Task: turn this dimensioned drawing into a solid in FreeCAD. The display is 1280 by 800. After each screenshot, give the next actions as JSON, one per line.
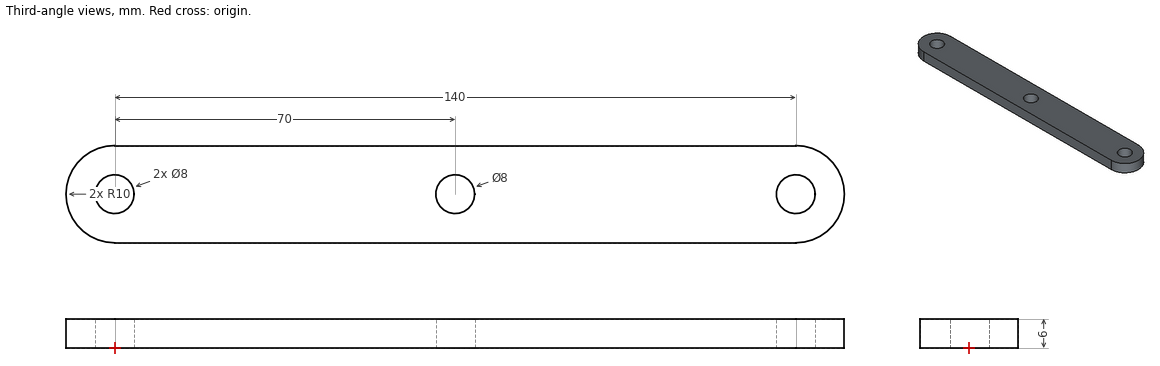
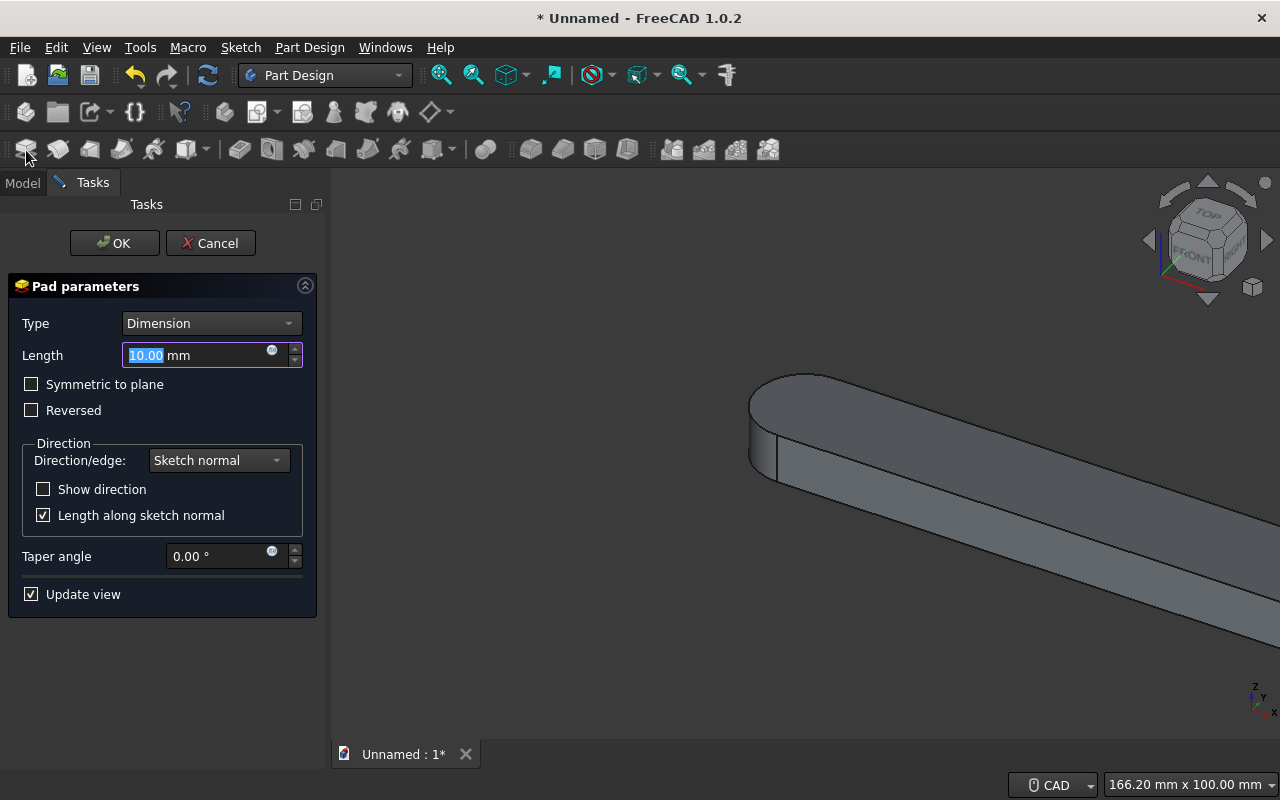
{"action": "type", "text": "6"}
{"action": "key", "text": "Tab"}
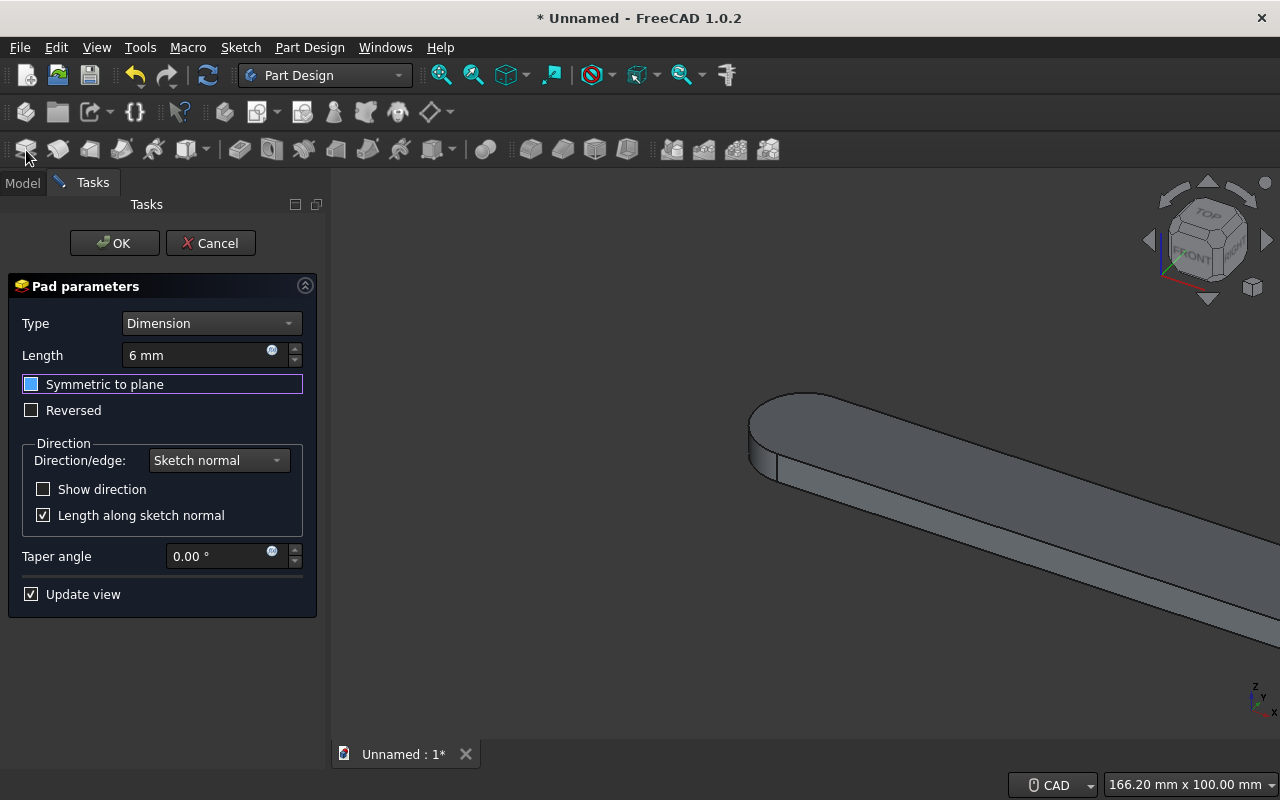
{"action": "left_click", "coordinate": [115, 243]}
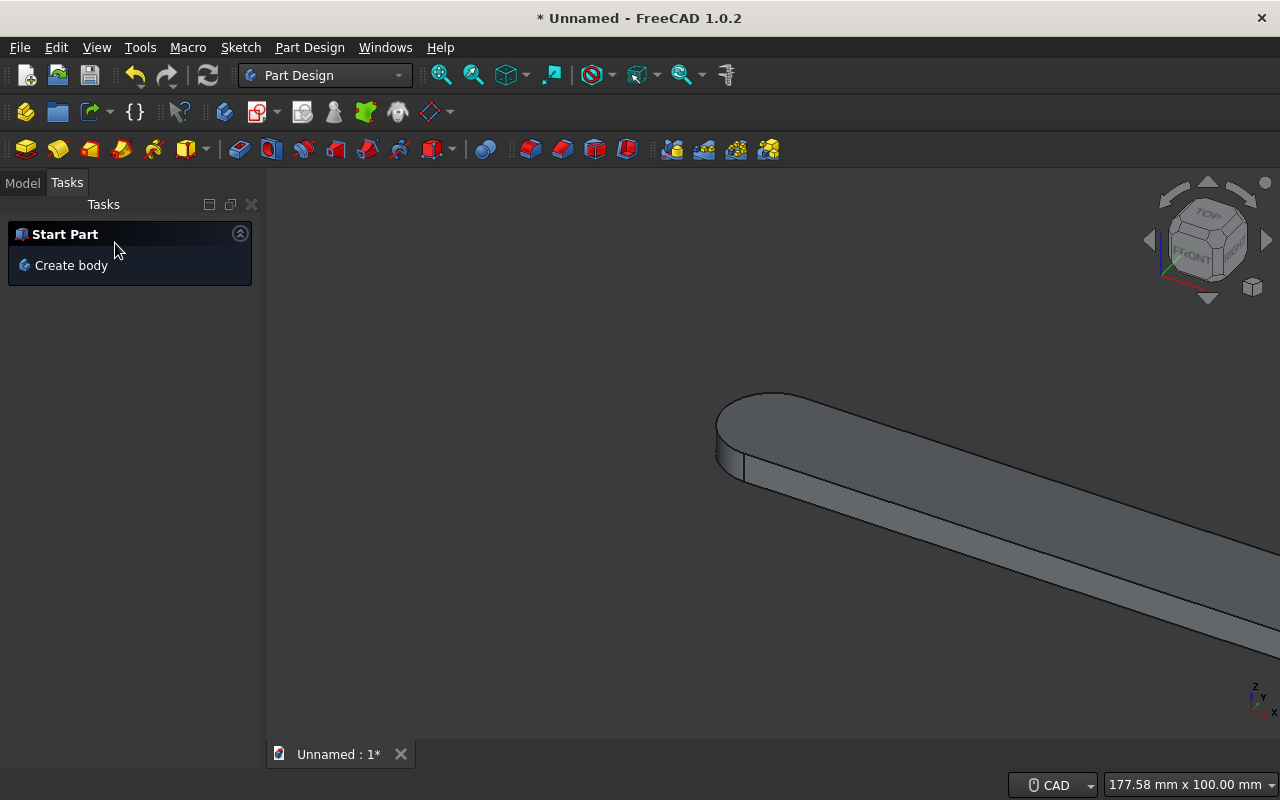
{"action": "left_click", "coordinate": [442, 76]}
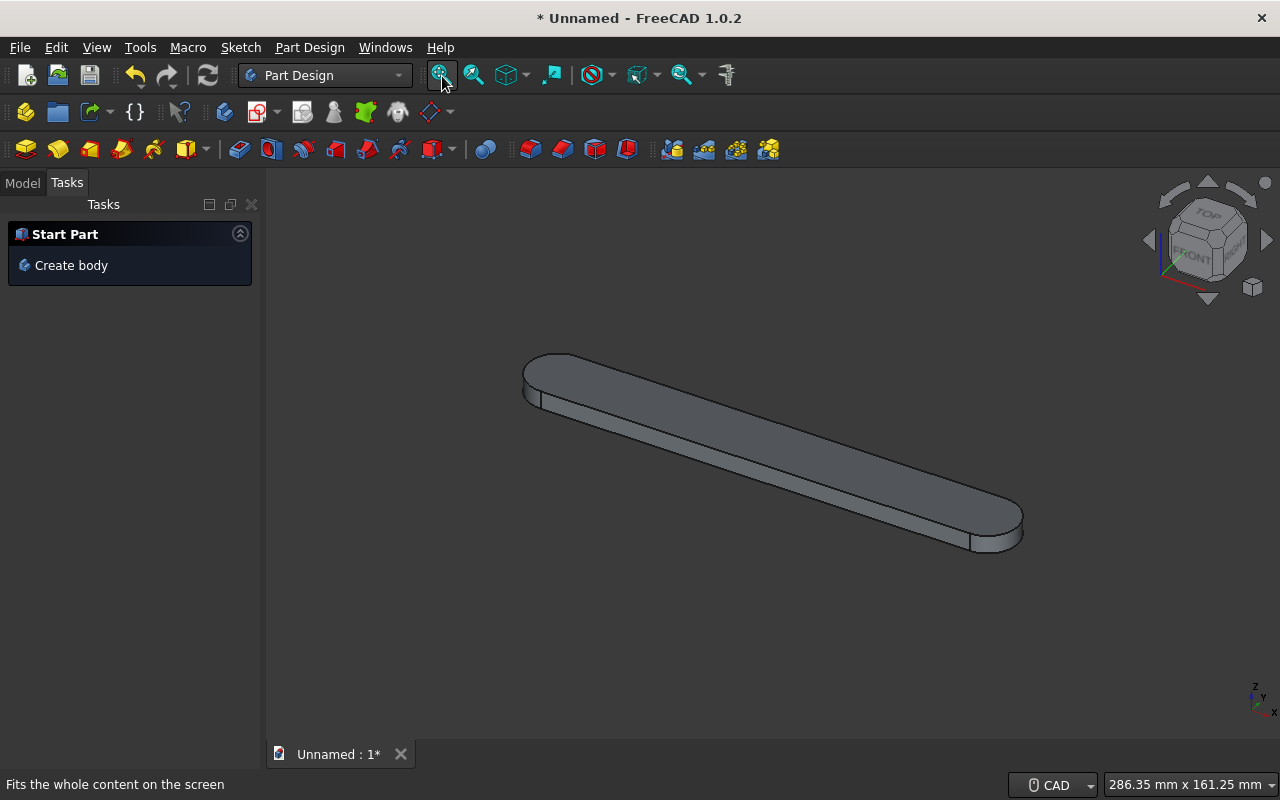
{"action": "left_click", "coordinate": [983, 513]}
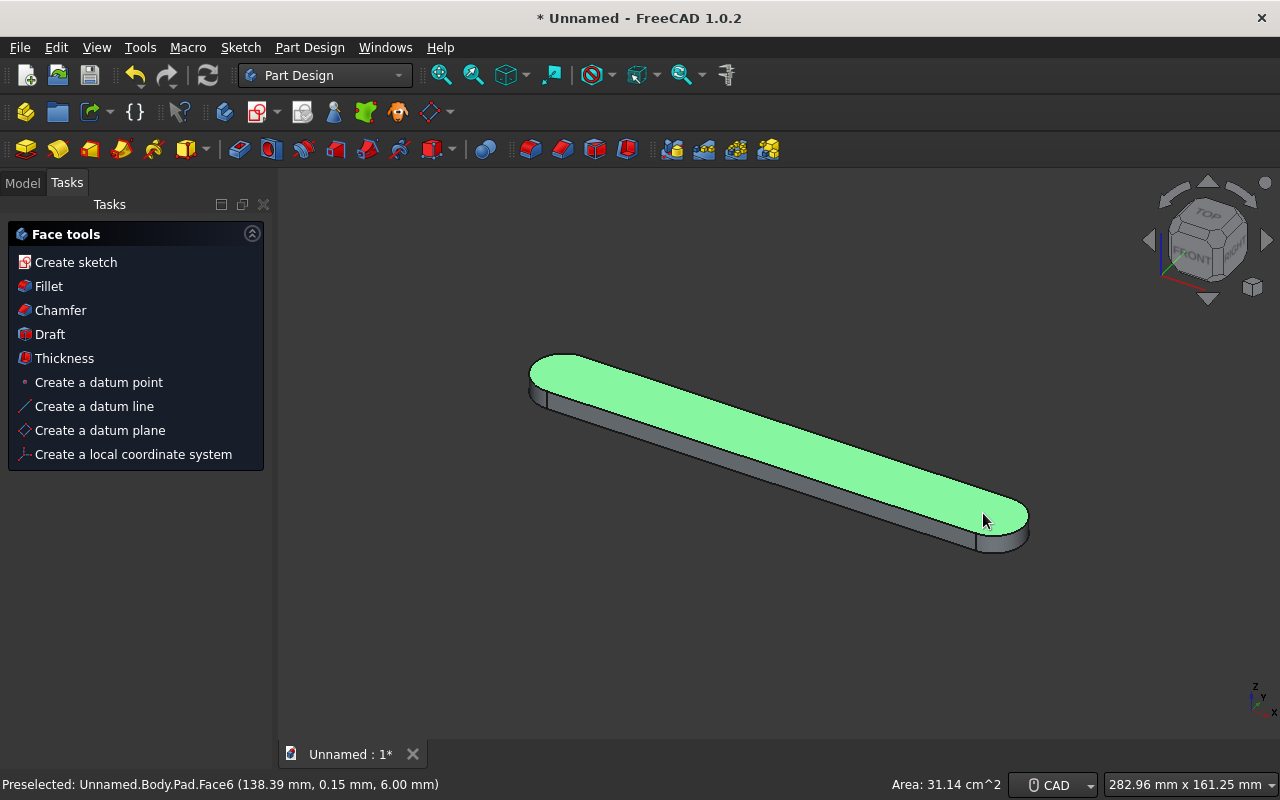
{"action": "left_click", "coordinate": [258, 112]}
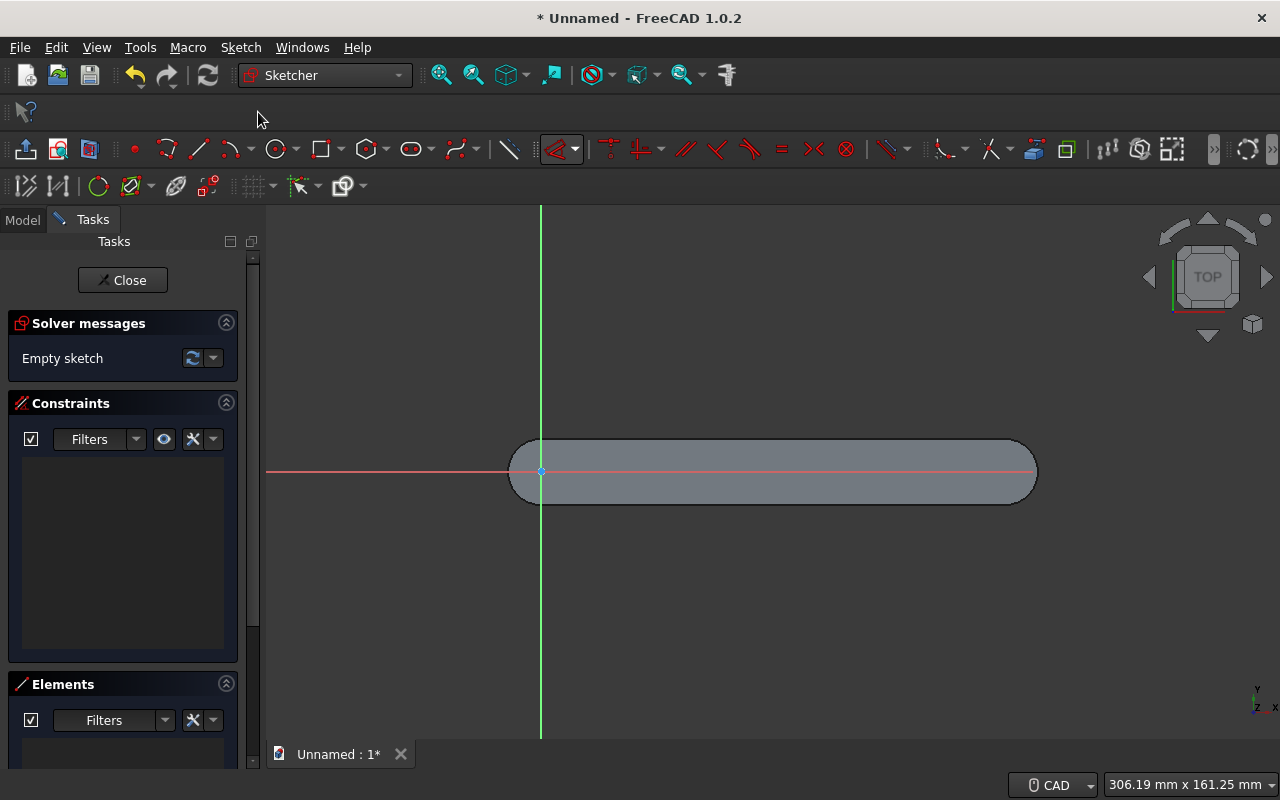
{"action": "left_click", "coordinate": [276, 150]}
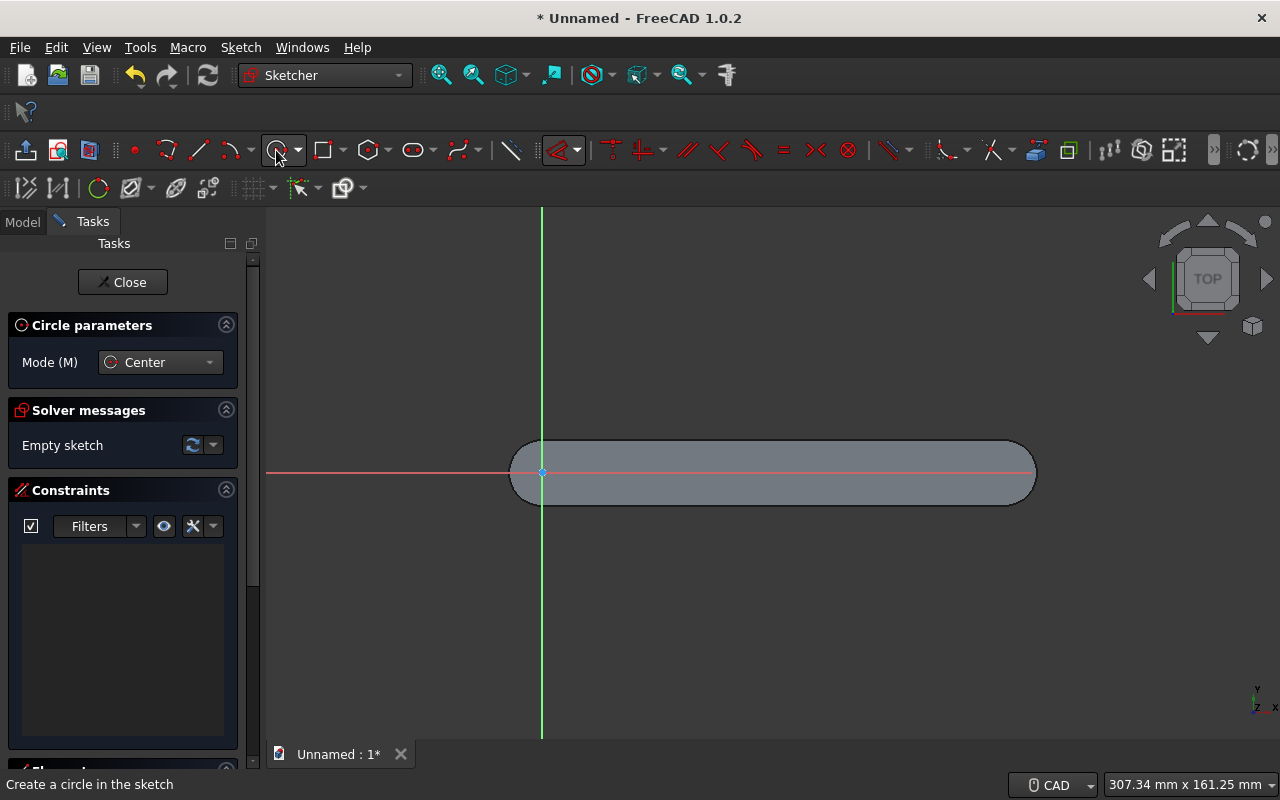
{"action": "scroll", "coordinate": [542, 473], "scroll_direction": "up", "scroll_amount": 3}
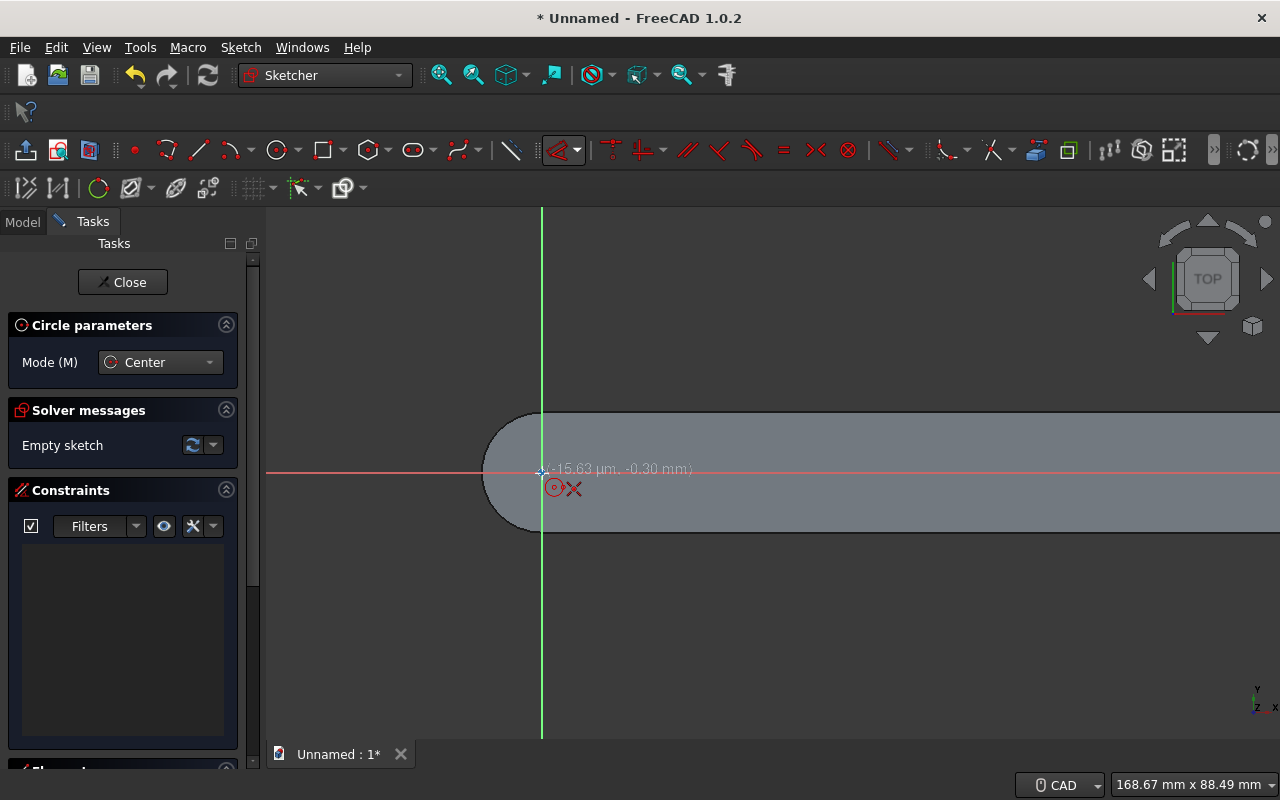
{"action": "left_click", "coordinate": [542, 473]}
{"action": "left_click", "coordinate": [559, 456]}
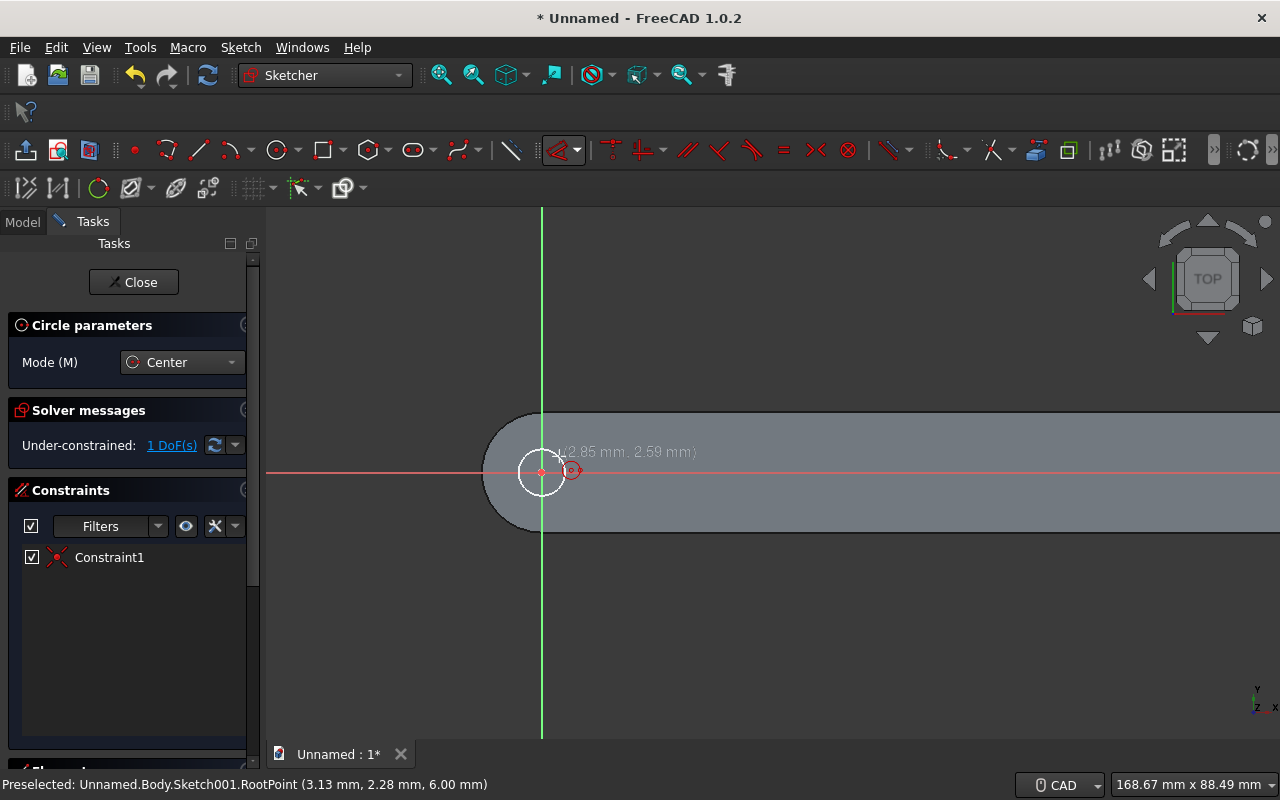
{"action": "scroll", "coordinate": [294, 474], "scroll_direction": "down", "scroll_amount": 2}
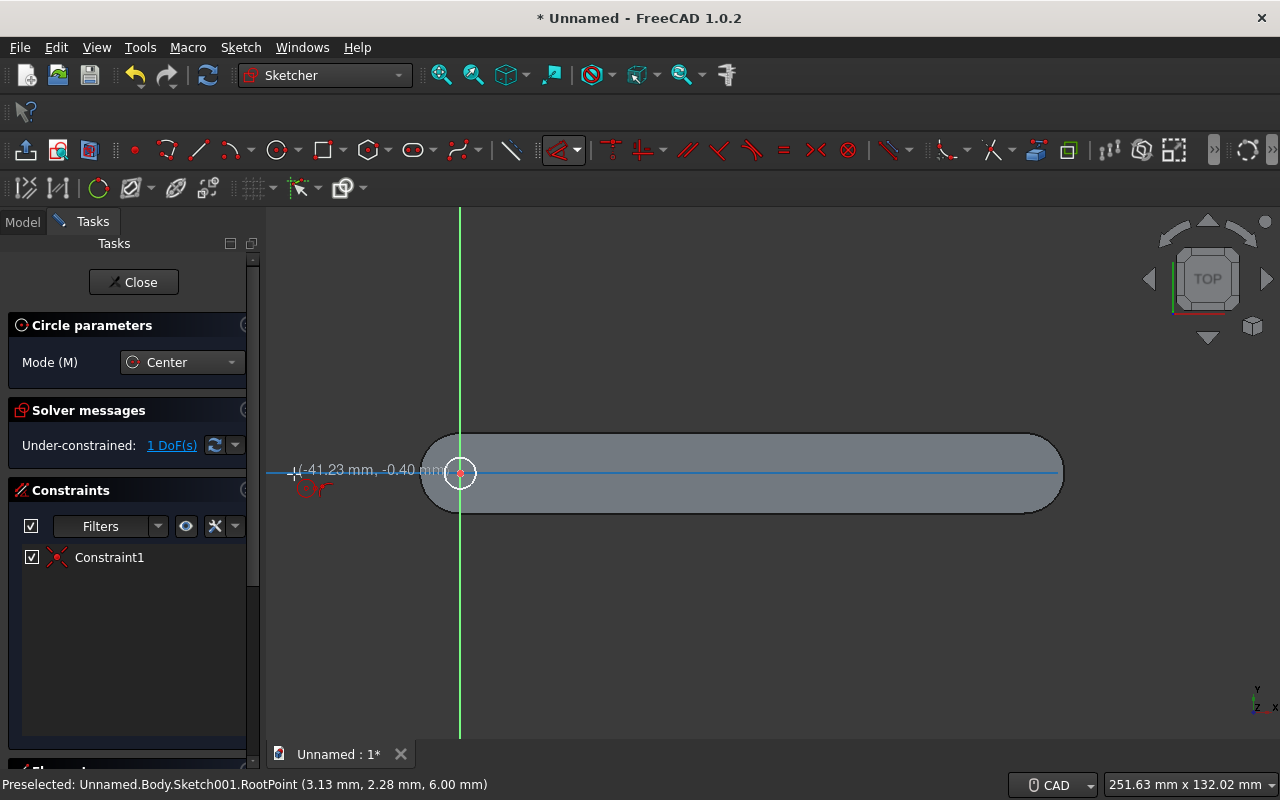
{"action": "scroll", "coordinate": [1024, 473], "scroll_direction": "up", "scroll_amount": 2}